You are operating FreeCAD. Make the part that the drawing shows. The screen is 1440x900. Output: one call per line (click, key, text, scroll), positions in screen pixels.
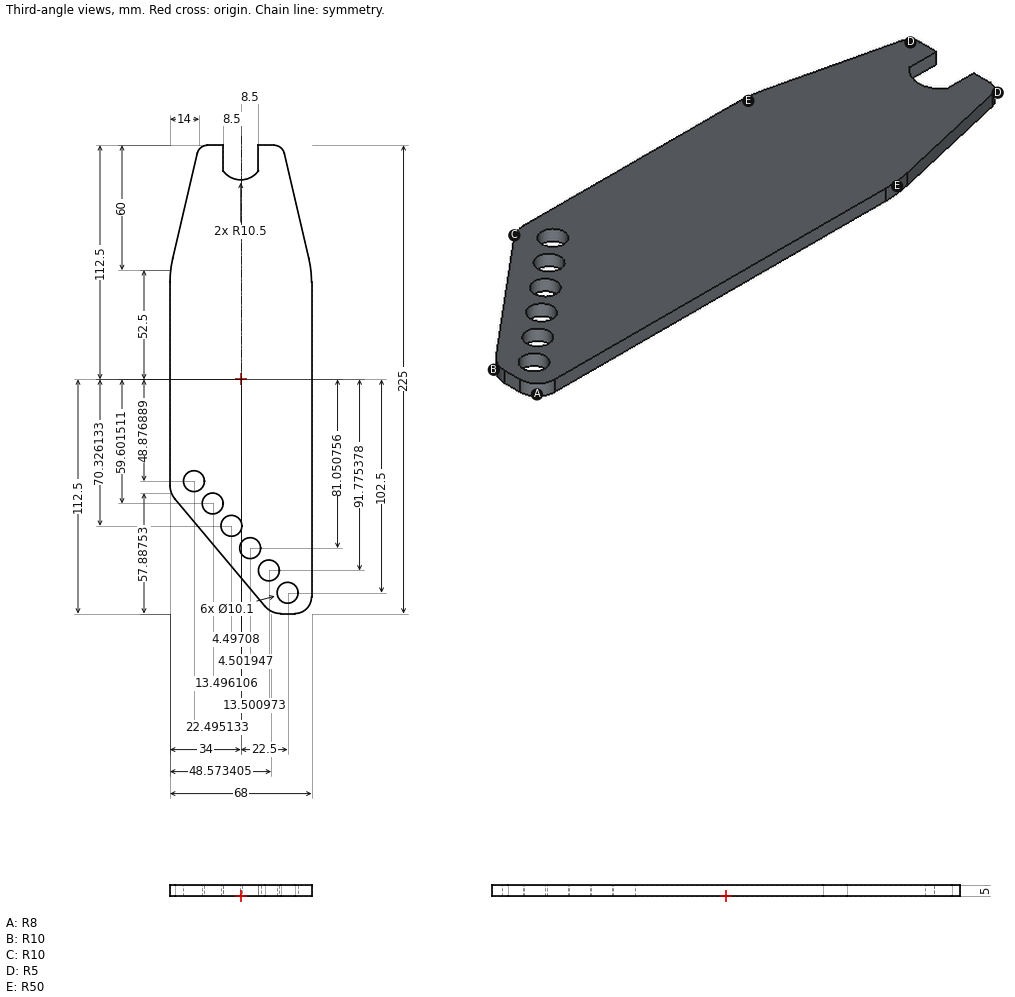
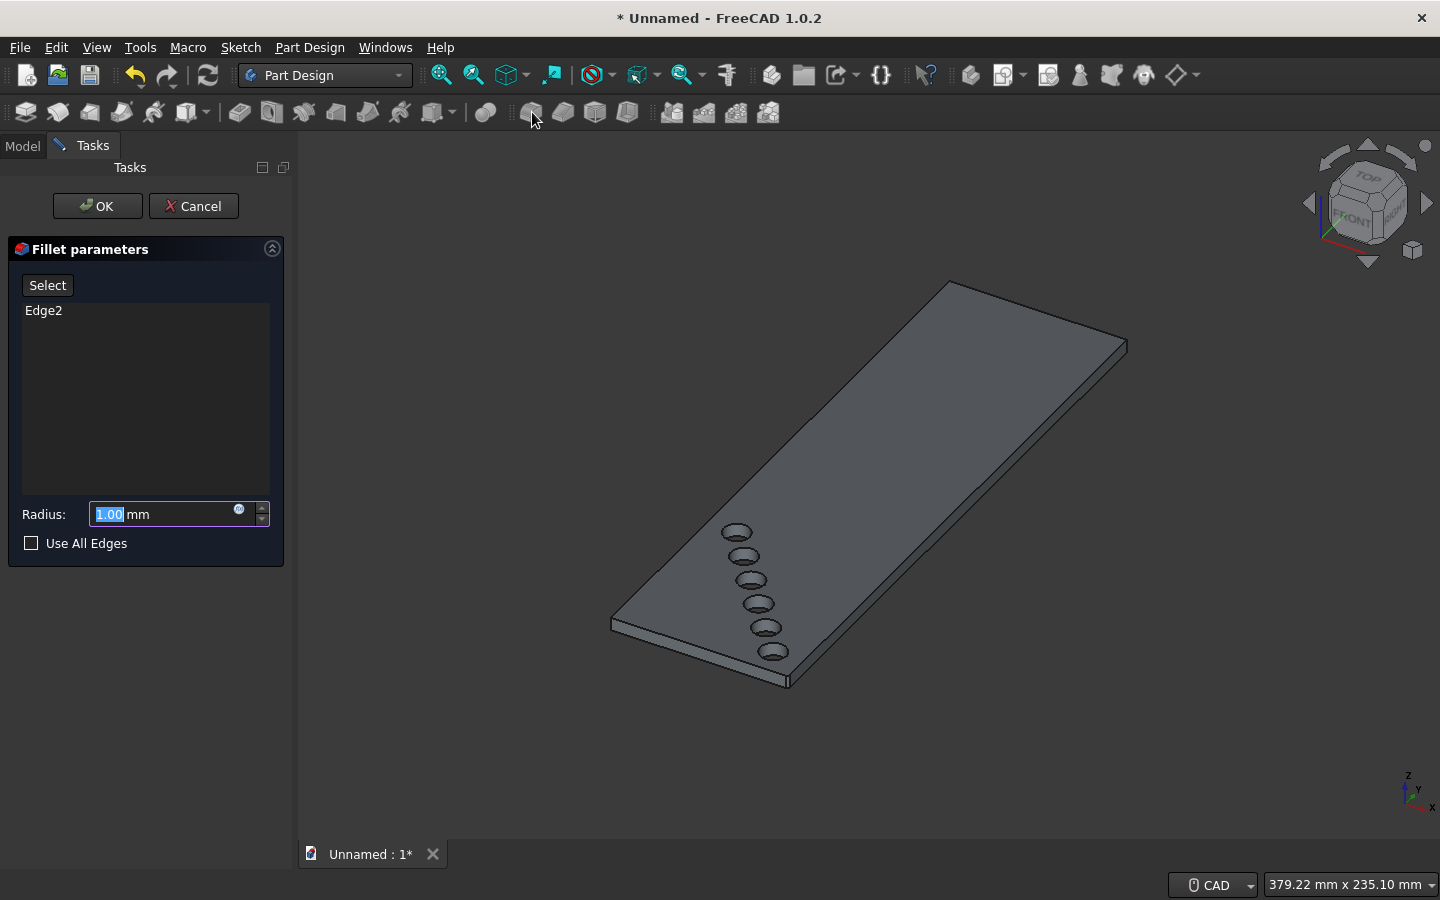
text(8)
key(Tab)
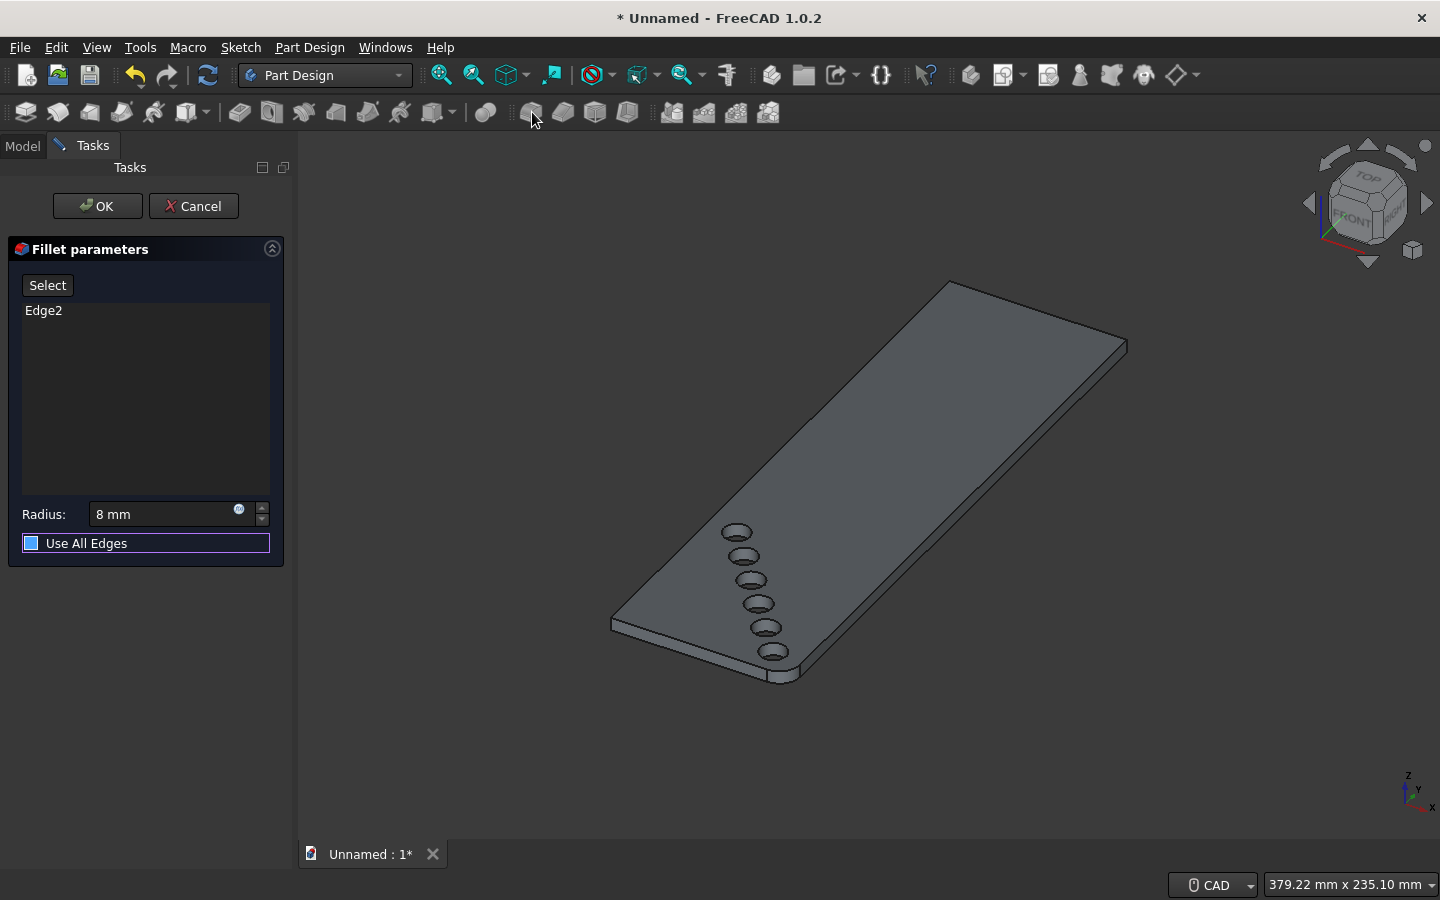
click(98, 206)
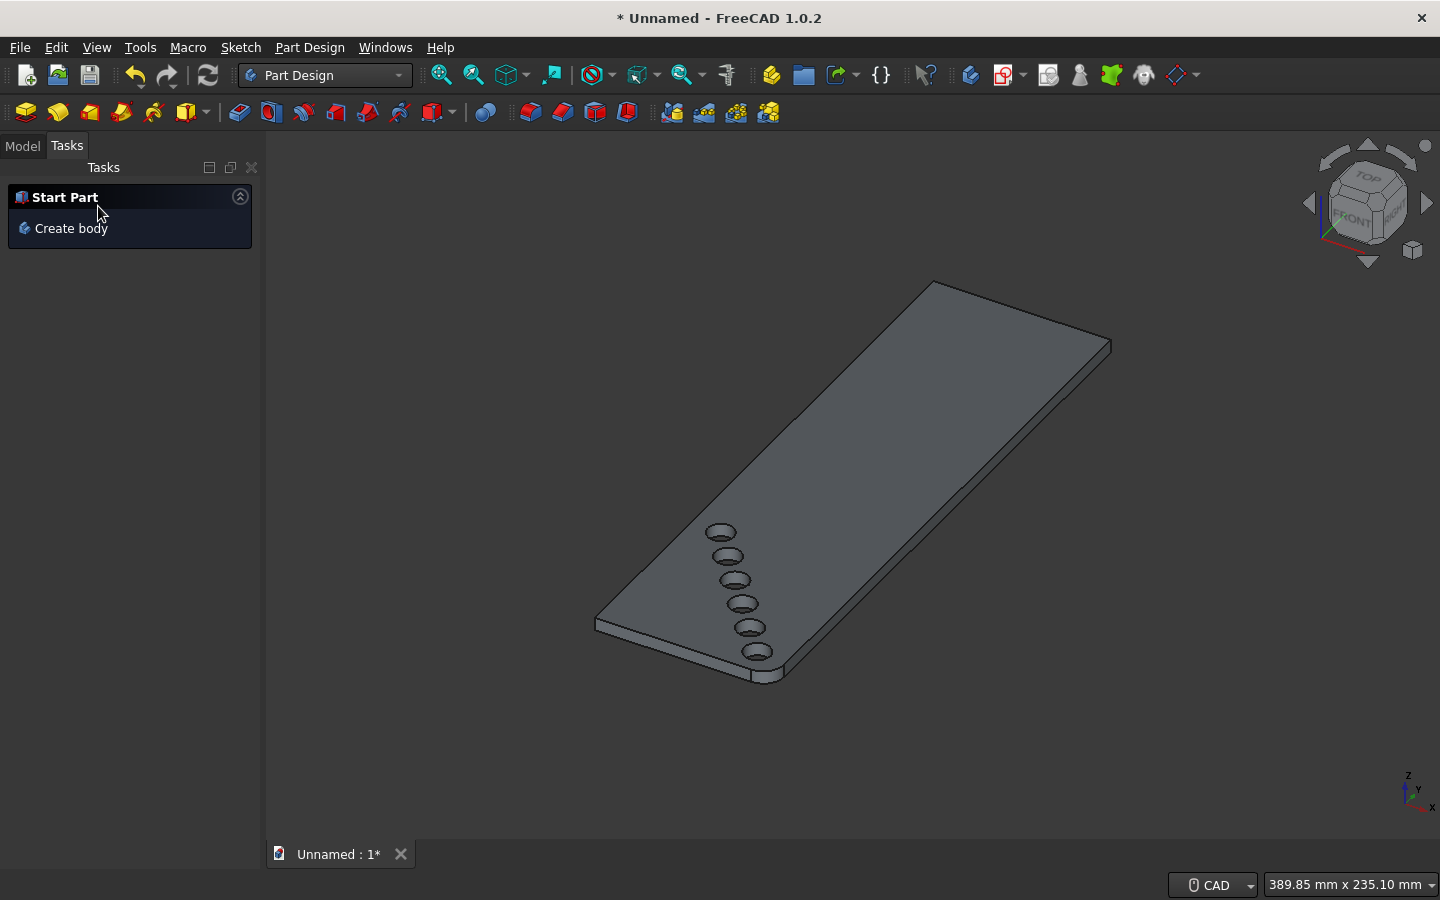
click(950, 382)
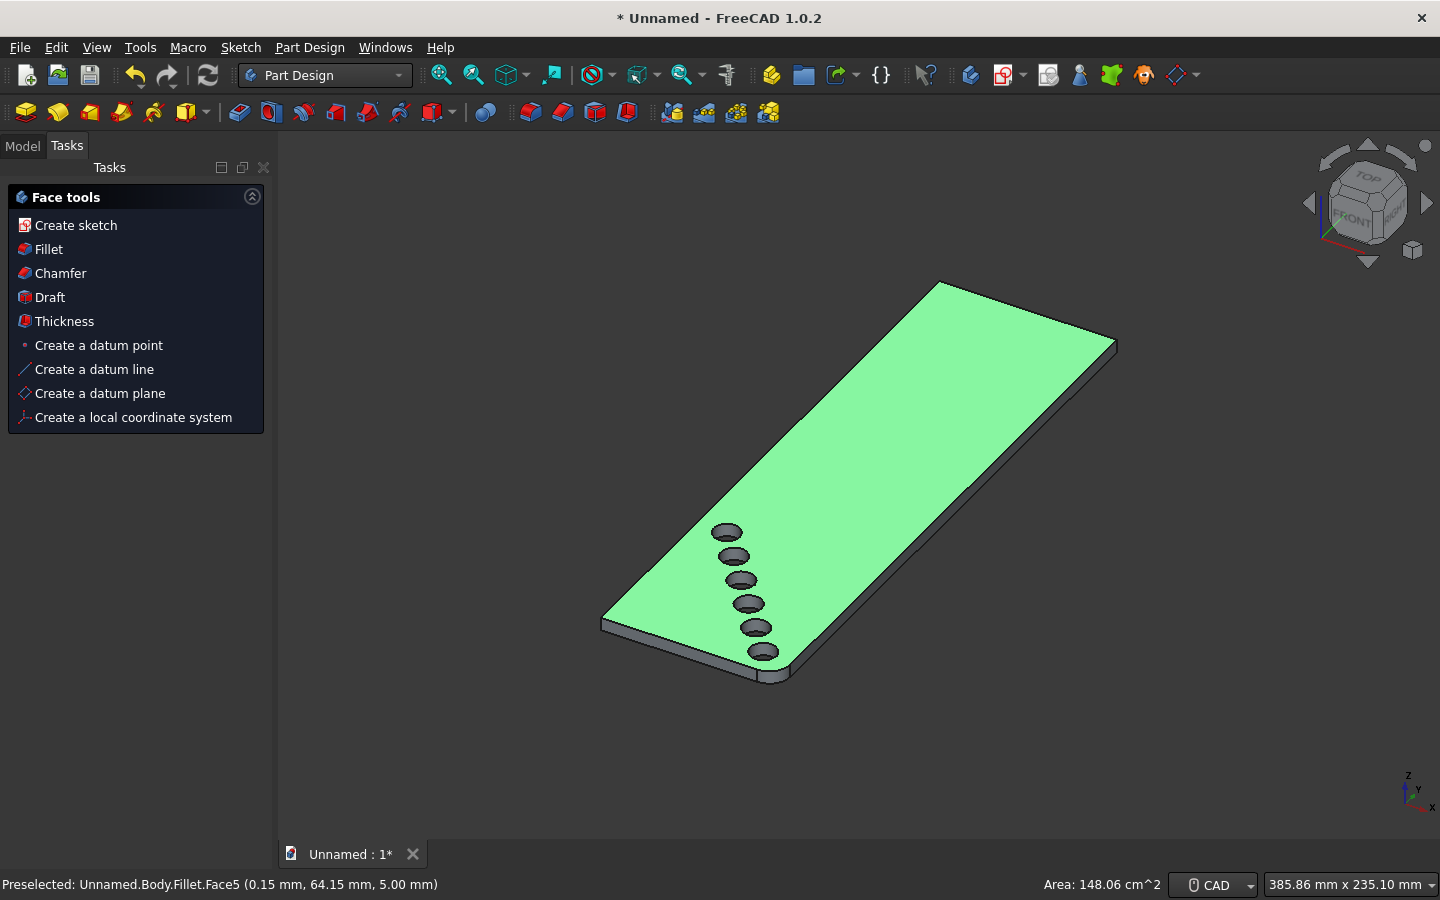
click(1004, 76)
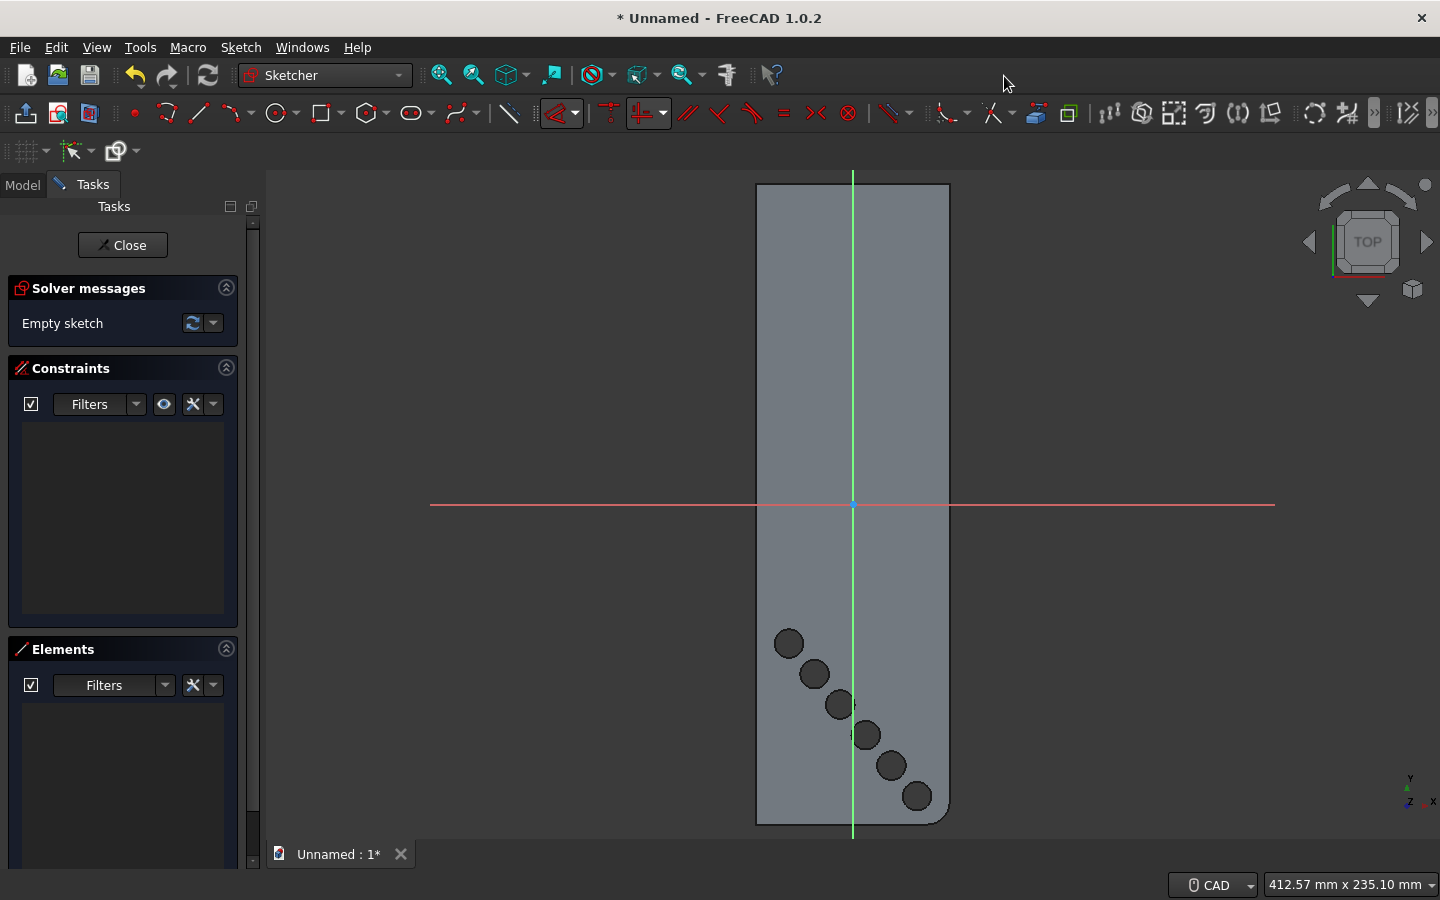
scroll(600, 198, down, 1)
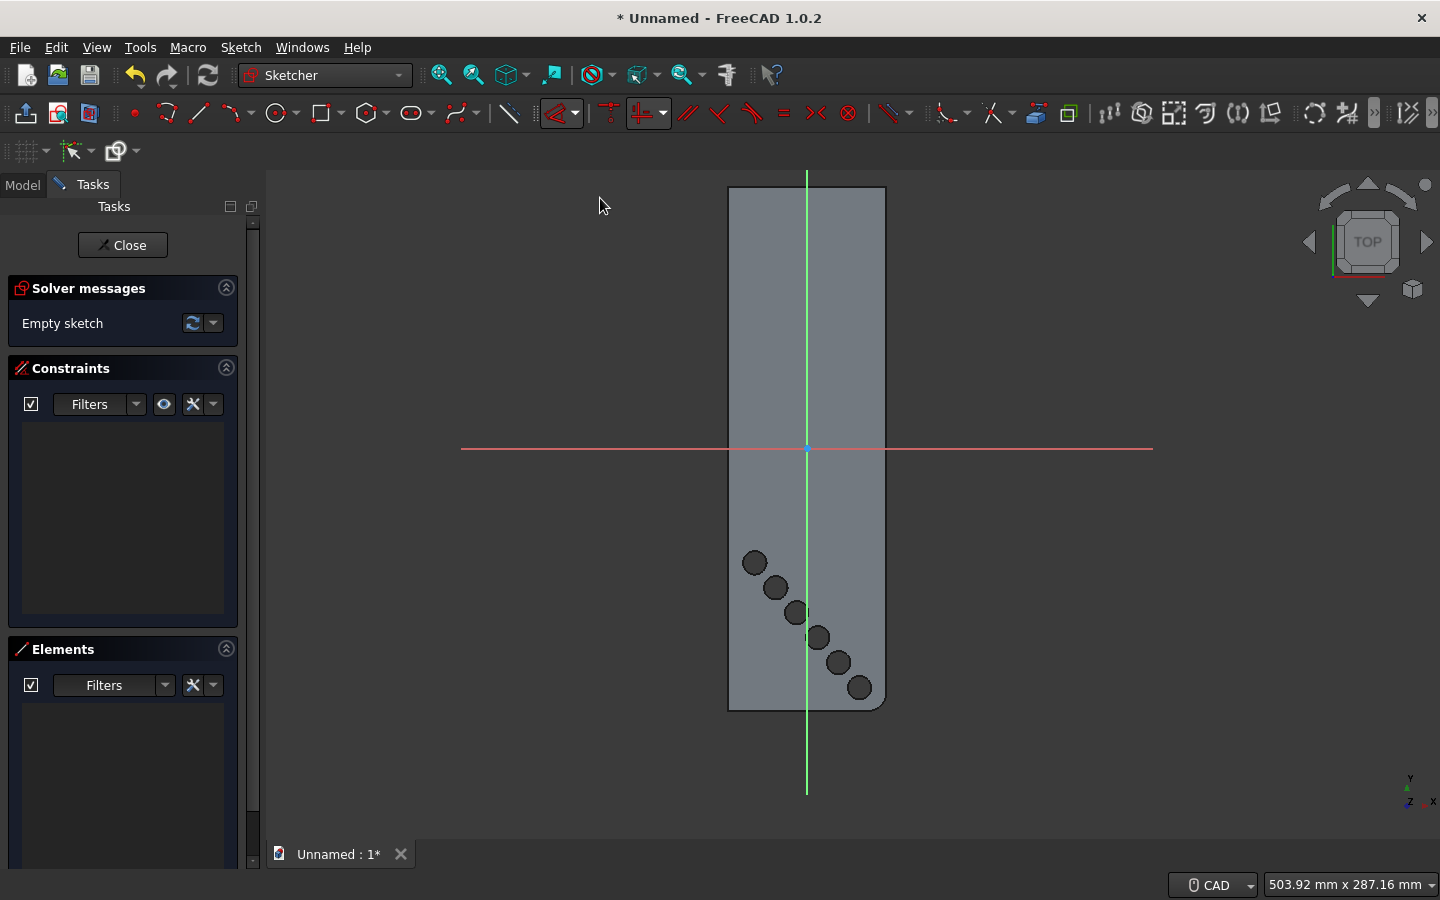
scroll(785, 672, up, 3)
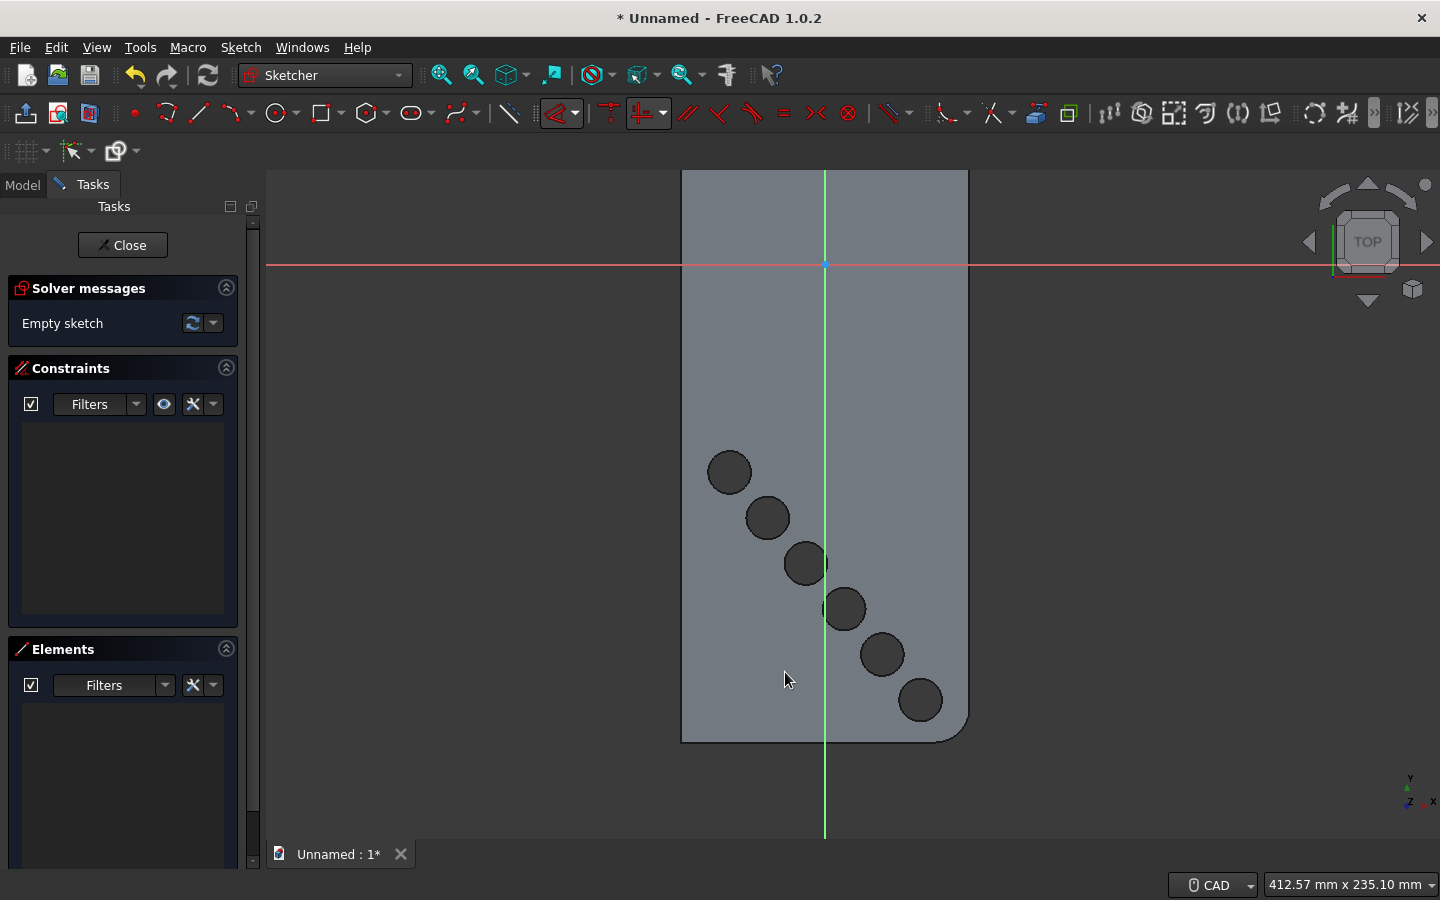
click(168, 114)